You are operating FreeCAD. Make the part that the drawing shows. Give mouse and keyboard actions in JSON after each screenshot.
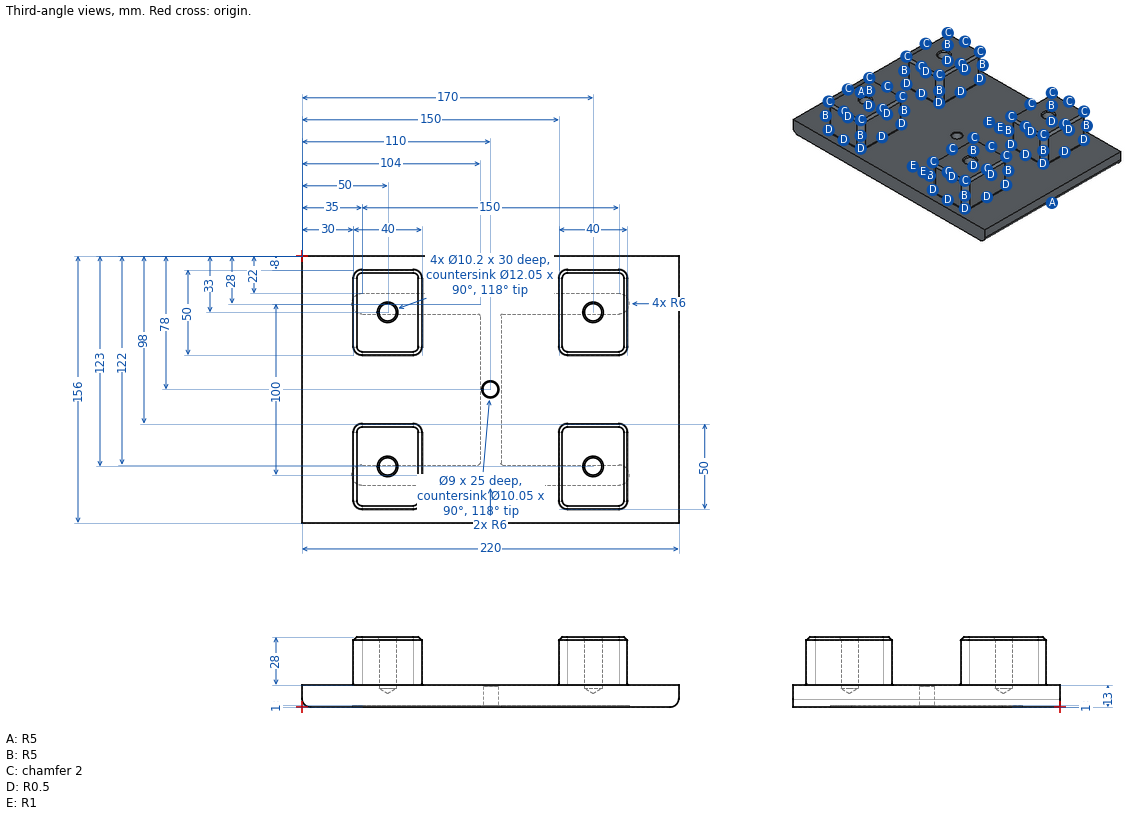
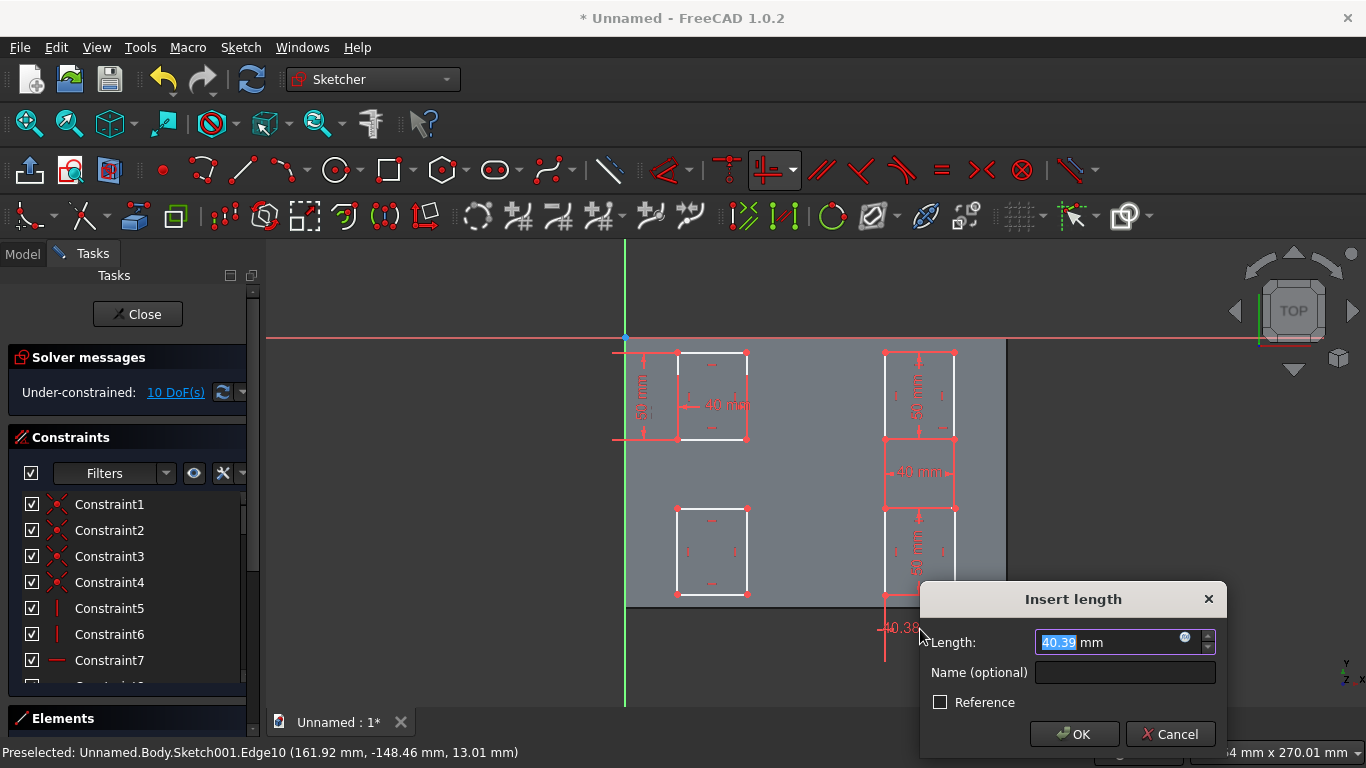
{"action": "type", "text": "40"}
{"action": "key", "text": "Return"}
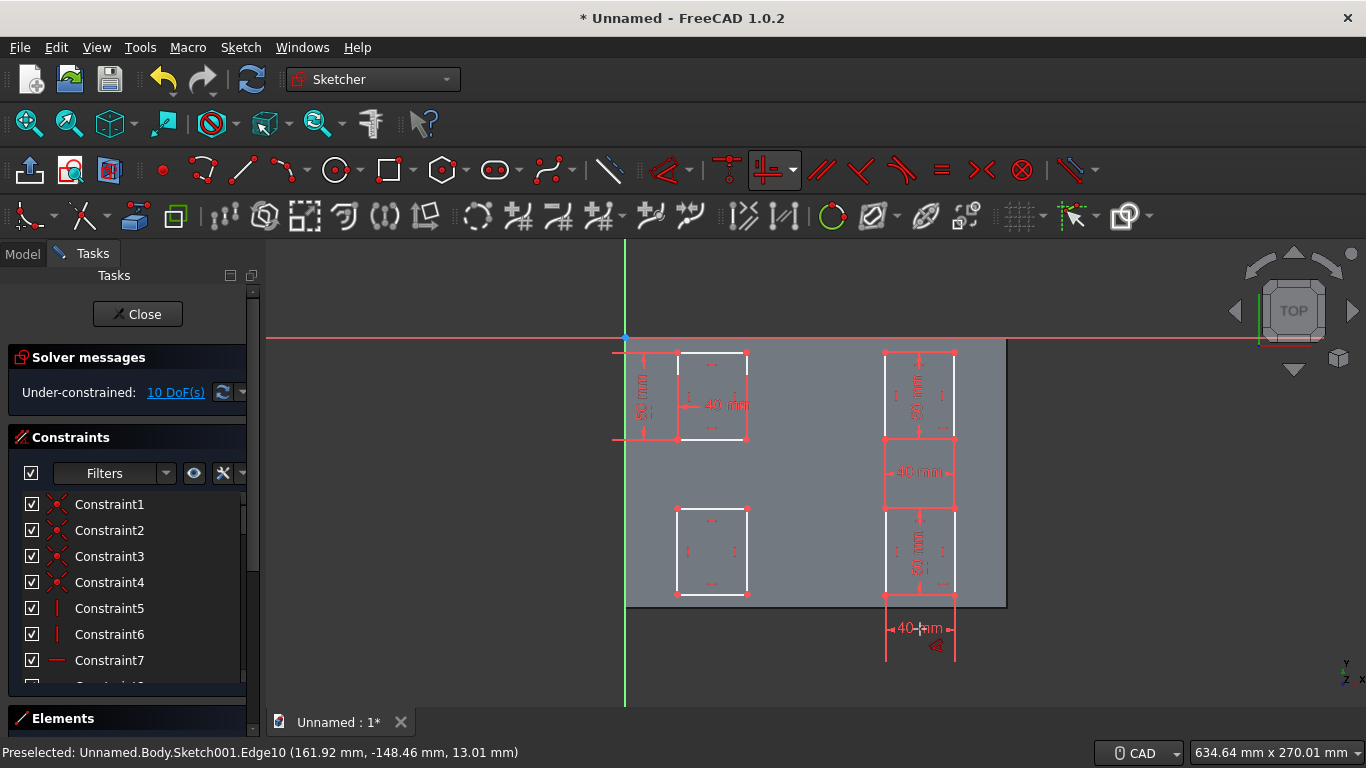
{"action": "left_click", "coordinate": [677, 535]}
{"action": "left_click", "coordinate": [643, 552]}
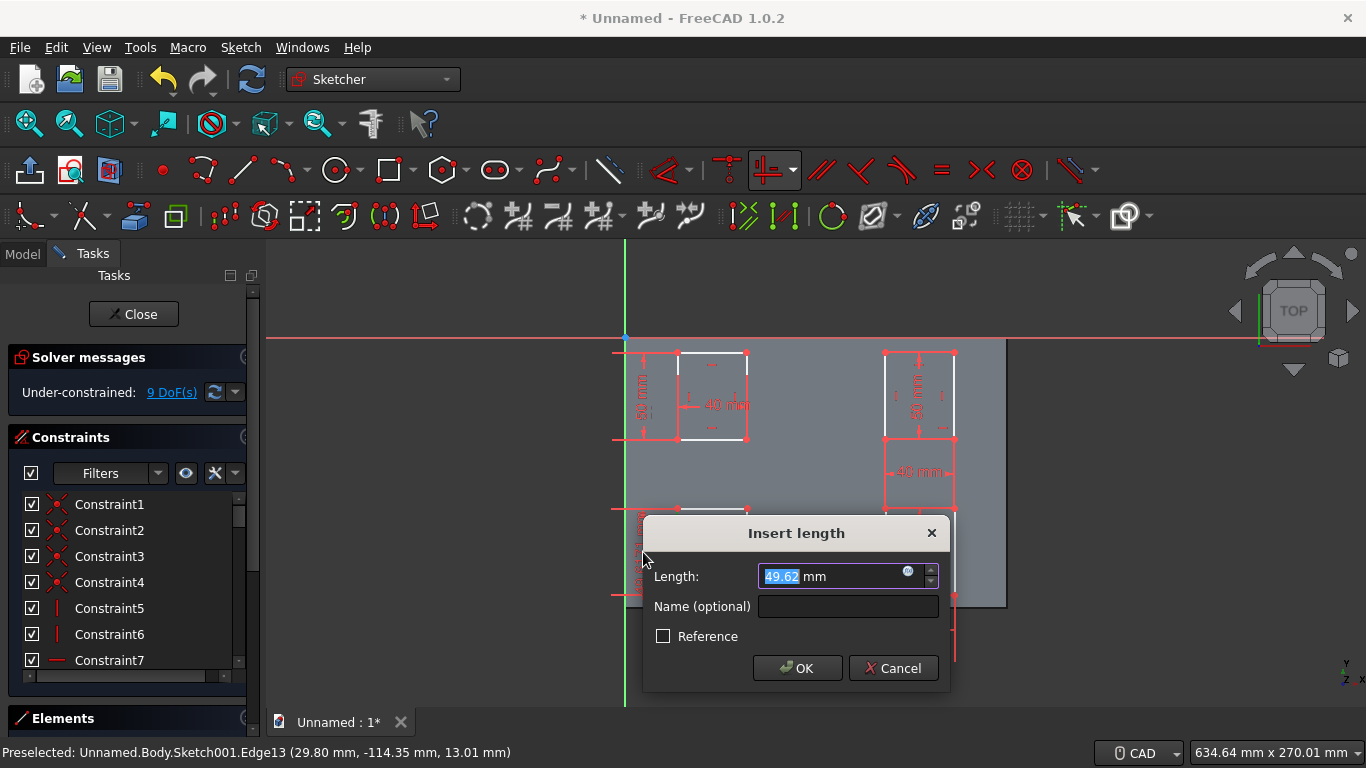
{"action": "type", "text": "50"}
{"action": "key", "text": "Return"}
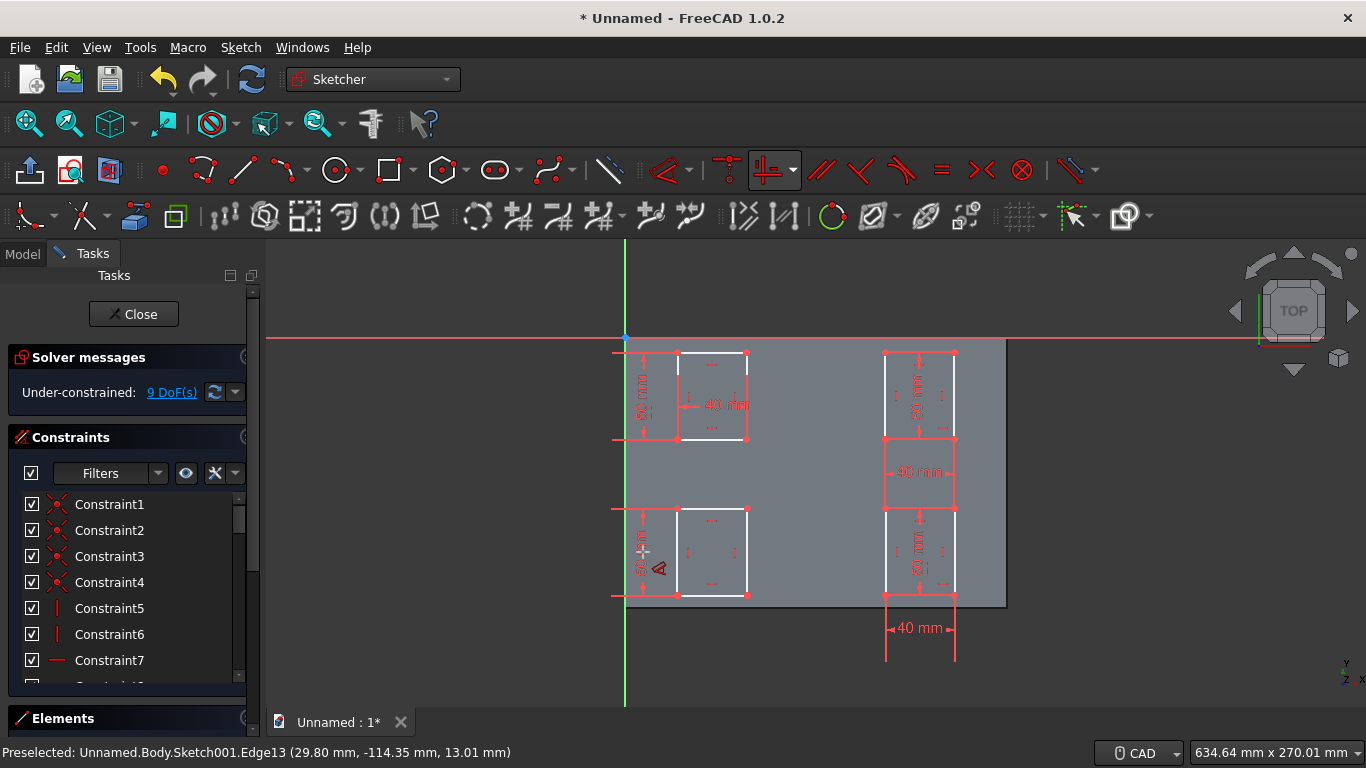
{"action": "left_click", "coordinate": [698, 596]}
{"action": "left_click", "coordinate": [712, 630]}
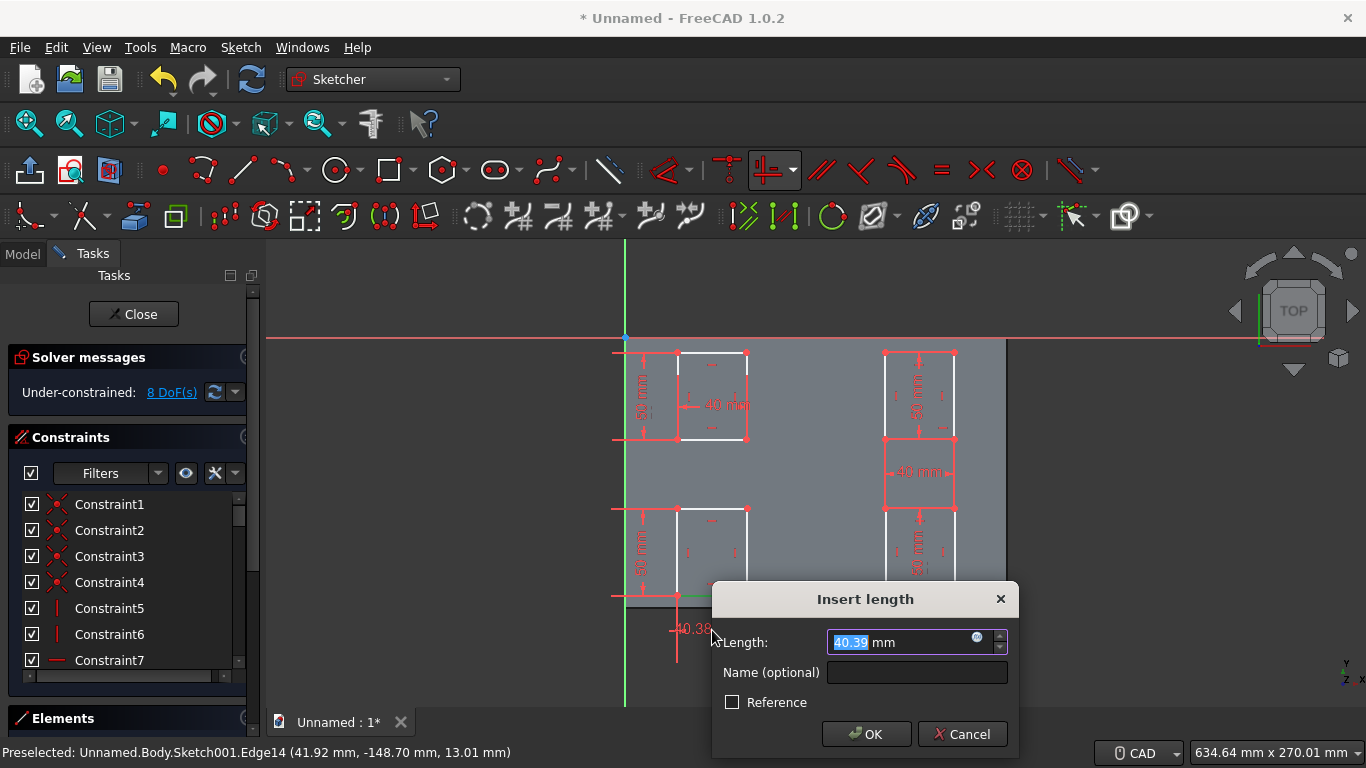
{"action": "type", "text": "40"}
{"action": "key", "text": "Return"}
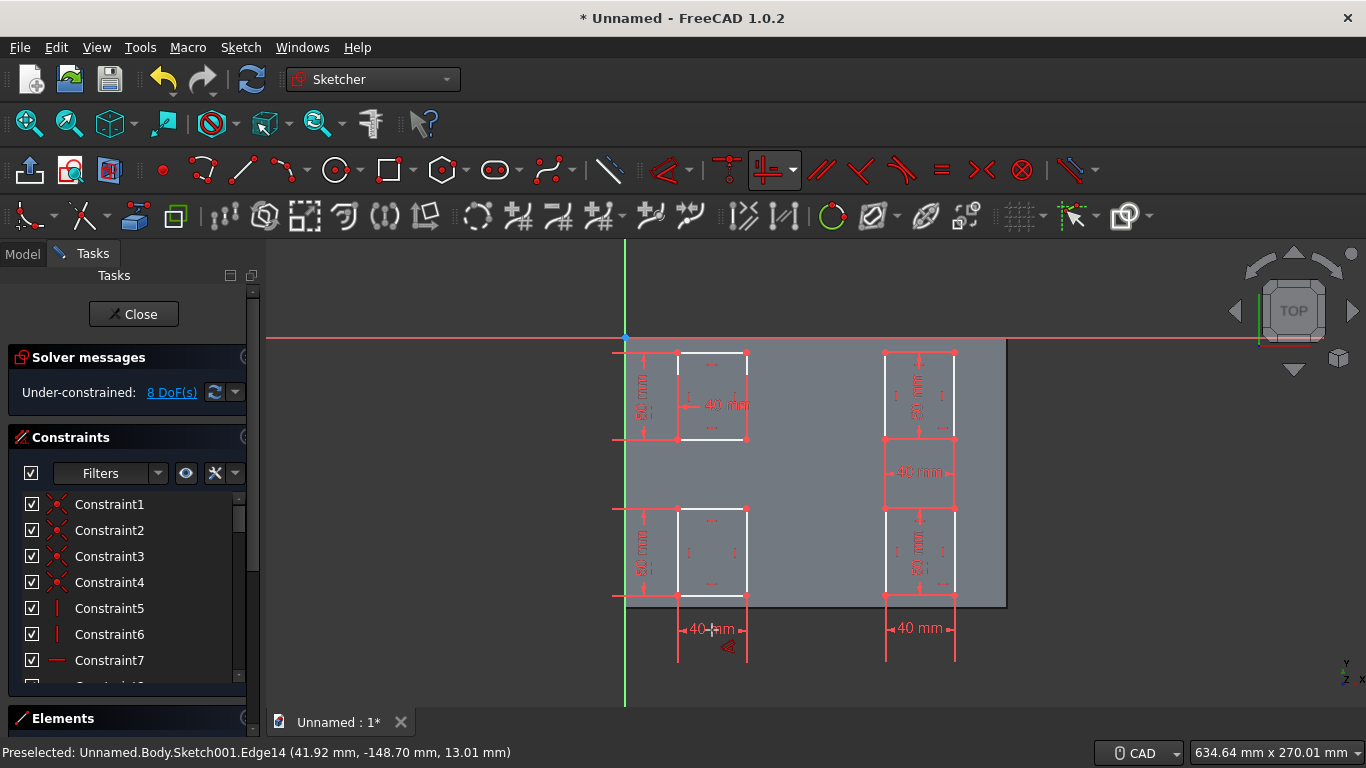
{"action": "scroll", "coordinate": [678, 353], "scroll_direction": "up", "scroll_amount": 6}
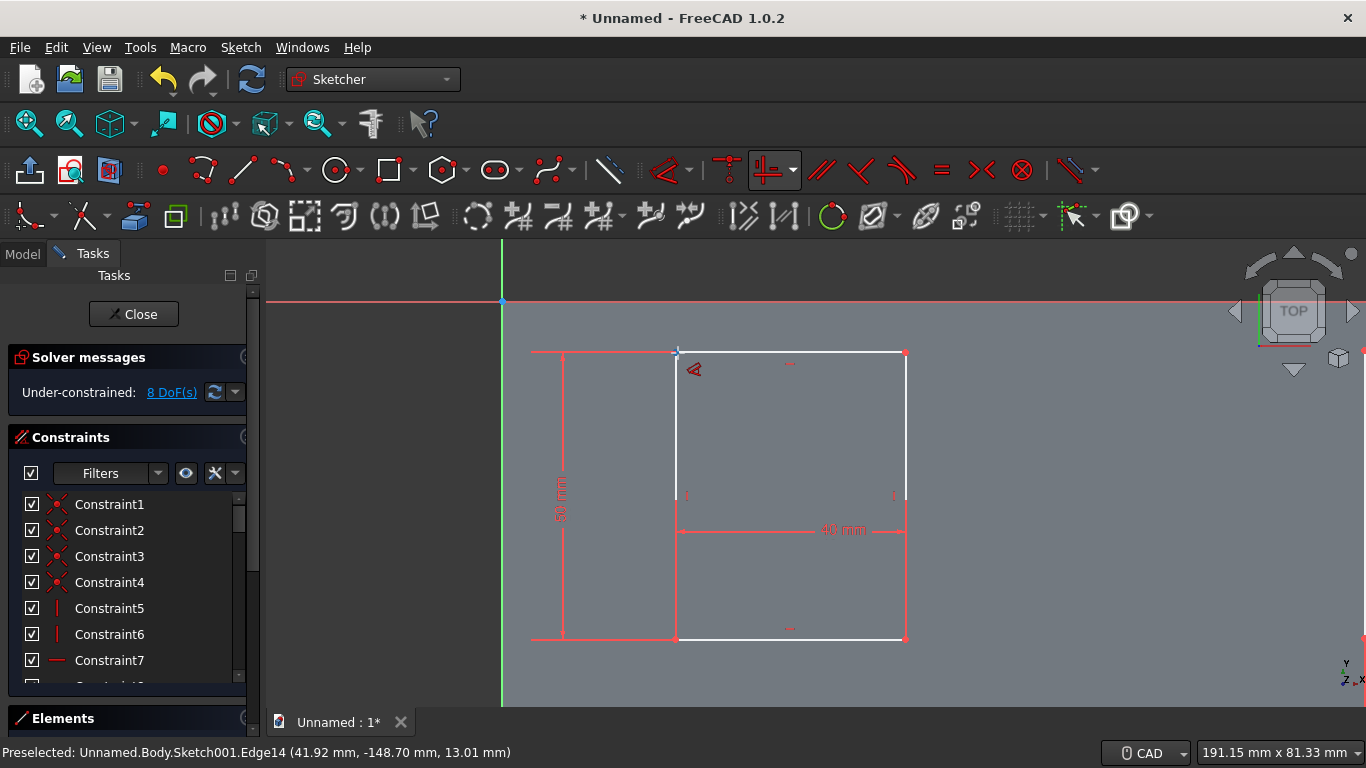
{"action": "left_click", "coordinate": [676, 352]}
{"action": "left_click", "coordinate": [468, 327]}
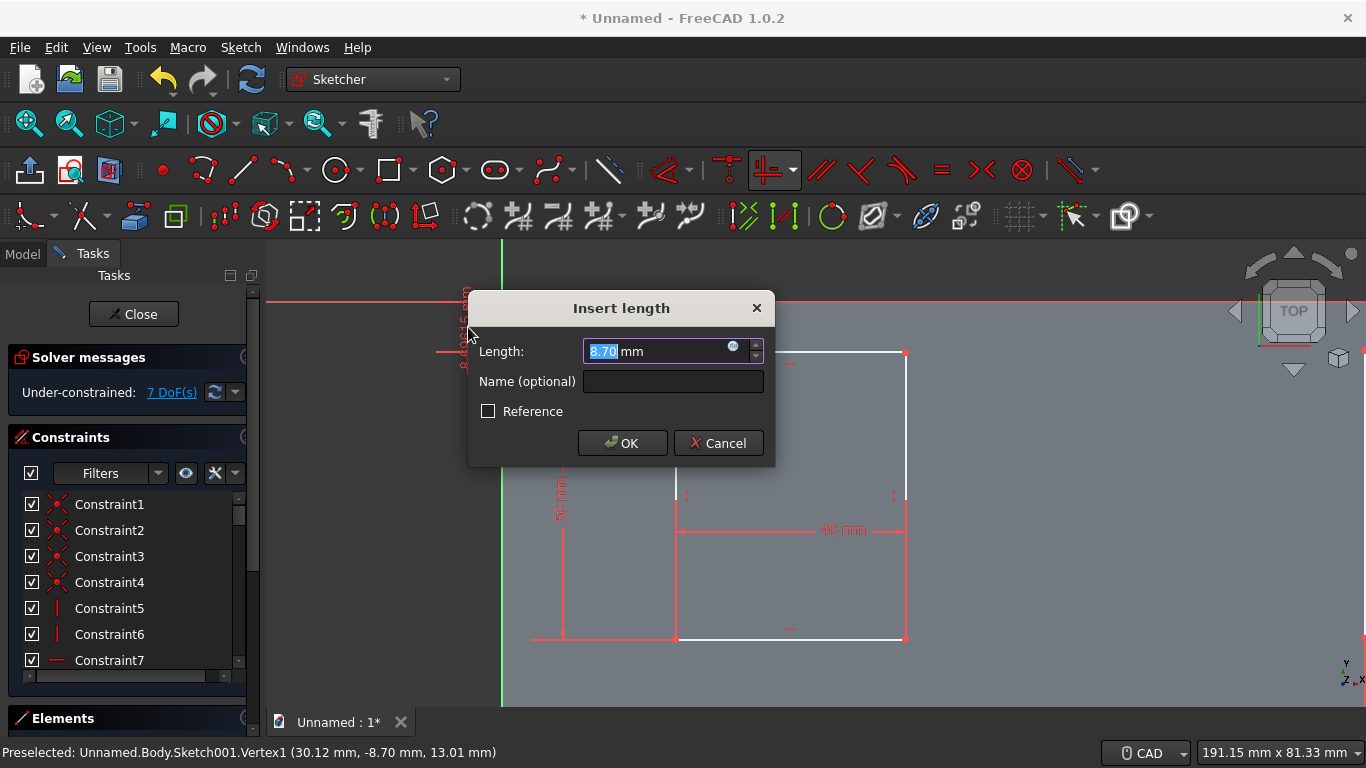
{"action": "type", "text": "8"}
{"action": "key", "text": "Return"}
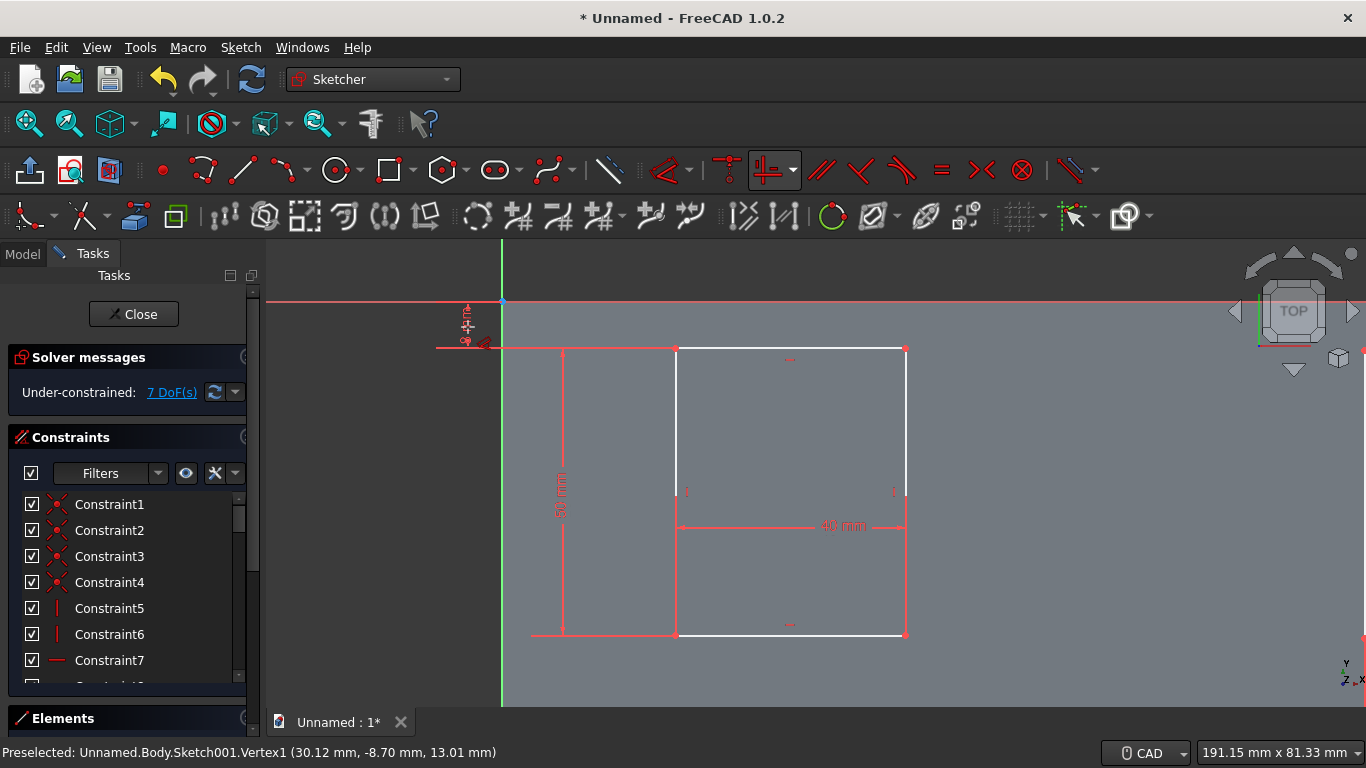
{"action": "scroll", "coordinate": [572, 325], "scroll_direction": "down", "scroll_amount": 5}